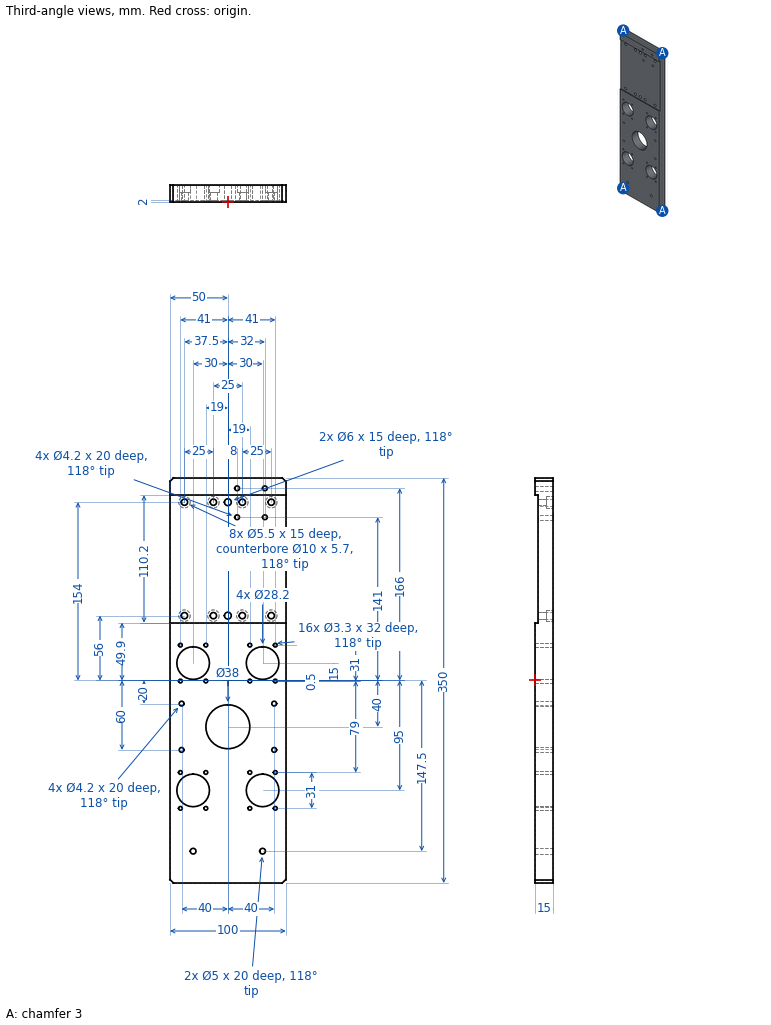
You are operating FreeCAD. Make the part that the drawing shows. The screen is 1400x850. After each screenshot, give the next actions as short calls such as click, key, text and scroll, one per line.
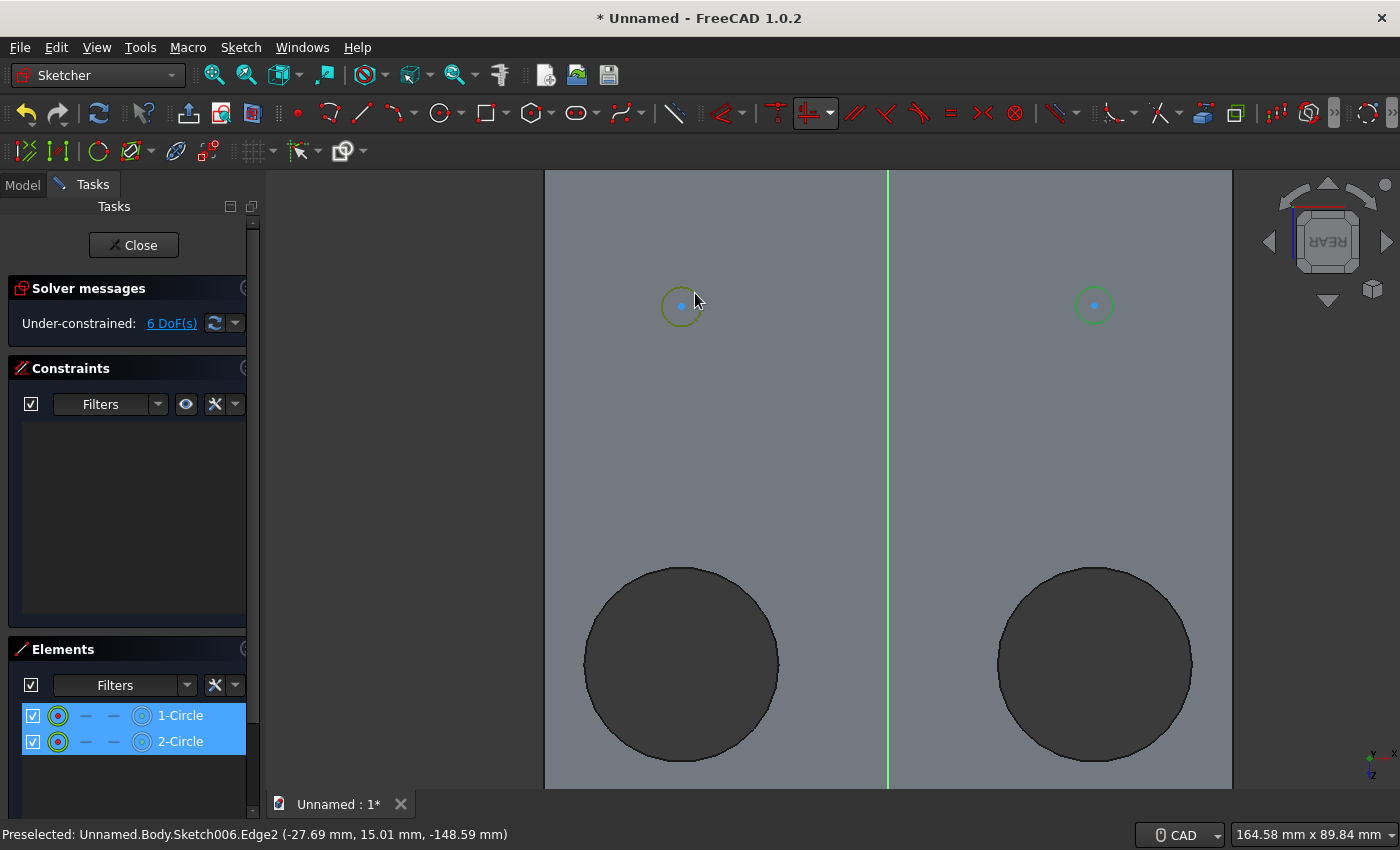
key(e)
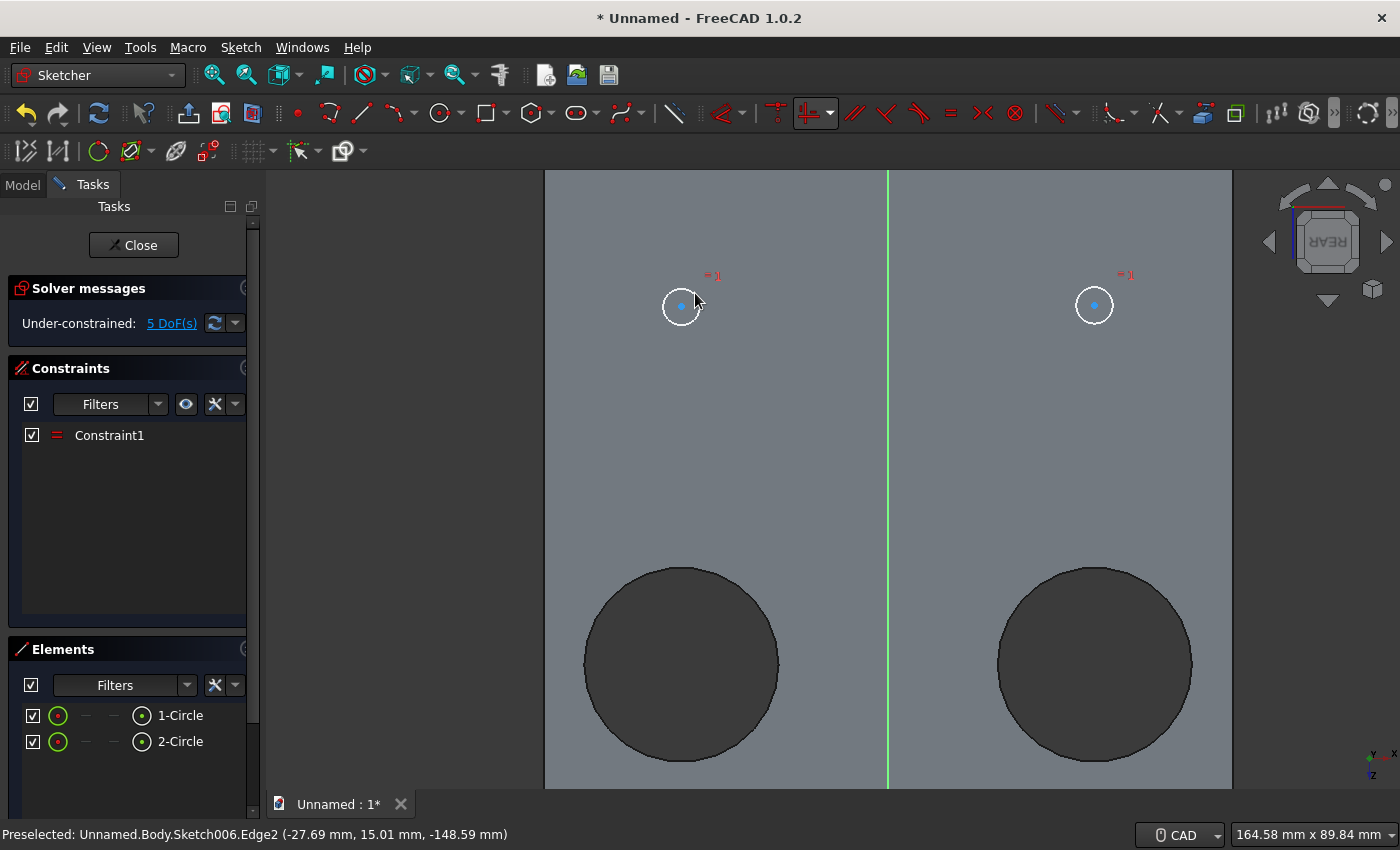
click(1094, 305)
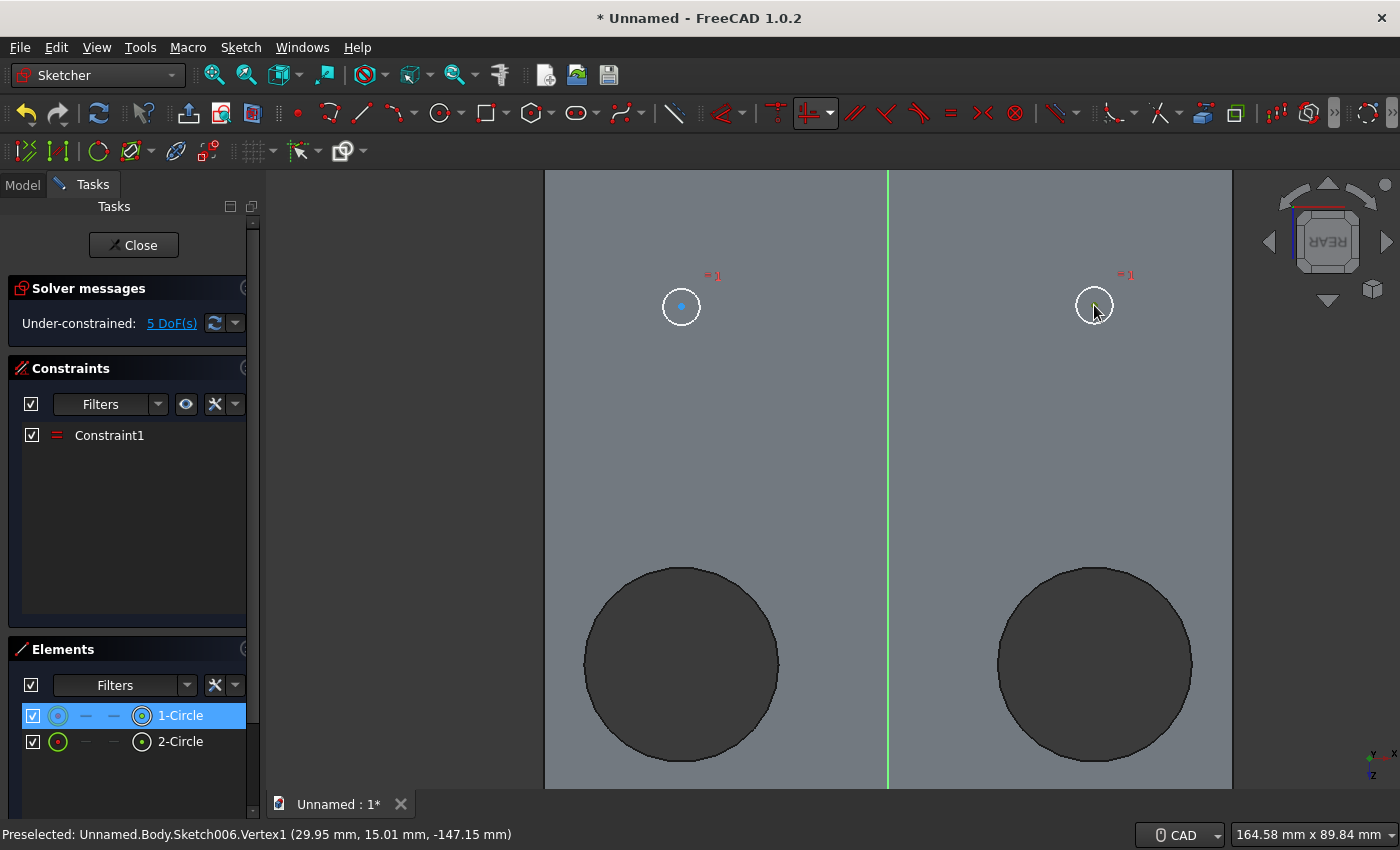
click(681, 307)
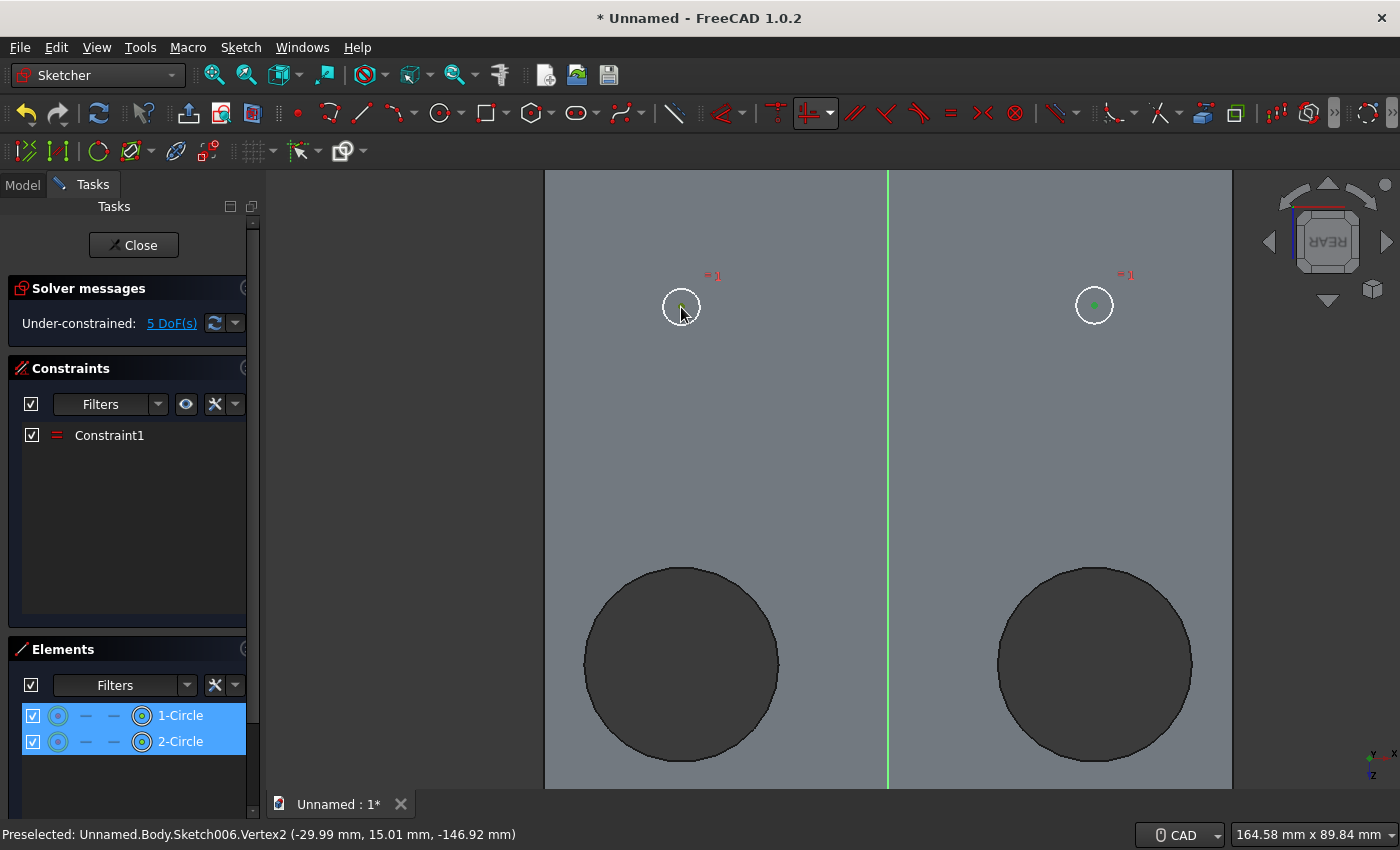
key(h)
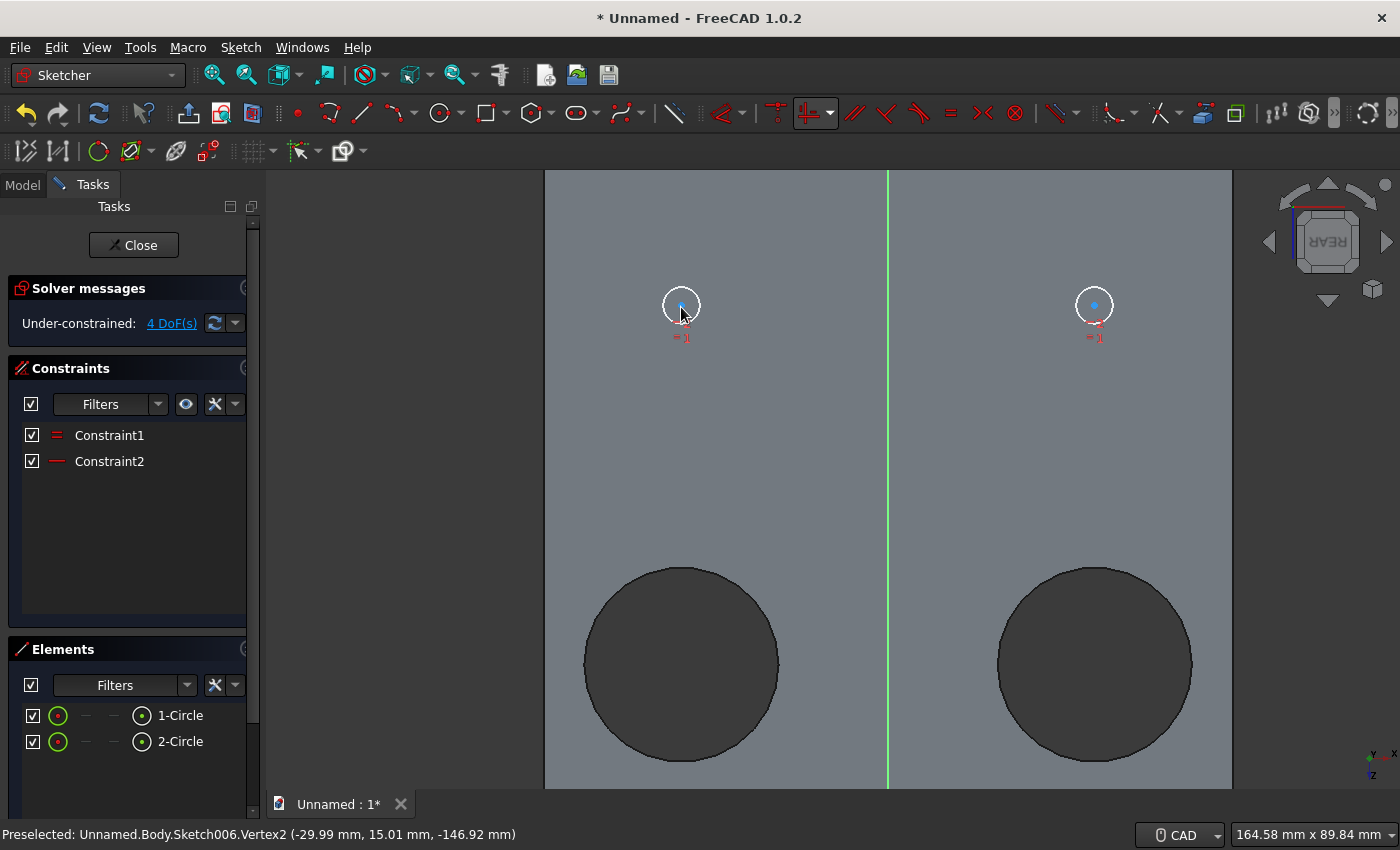
click(722, 114)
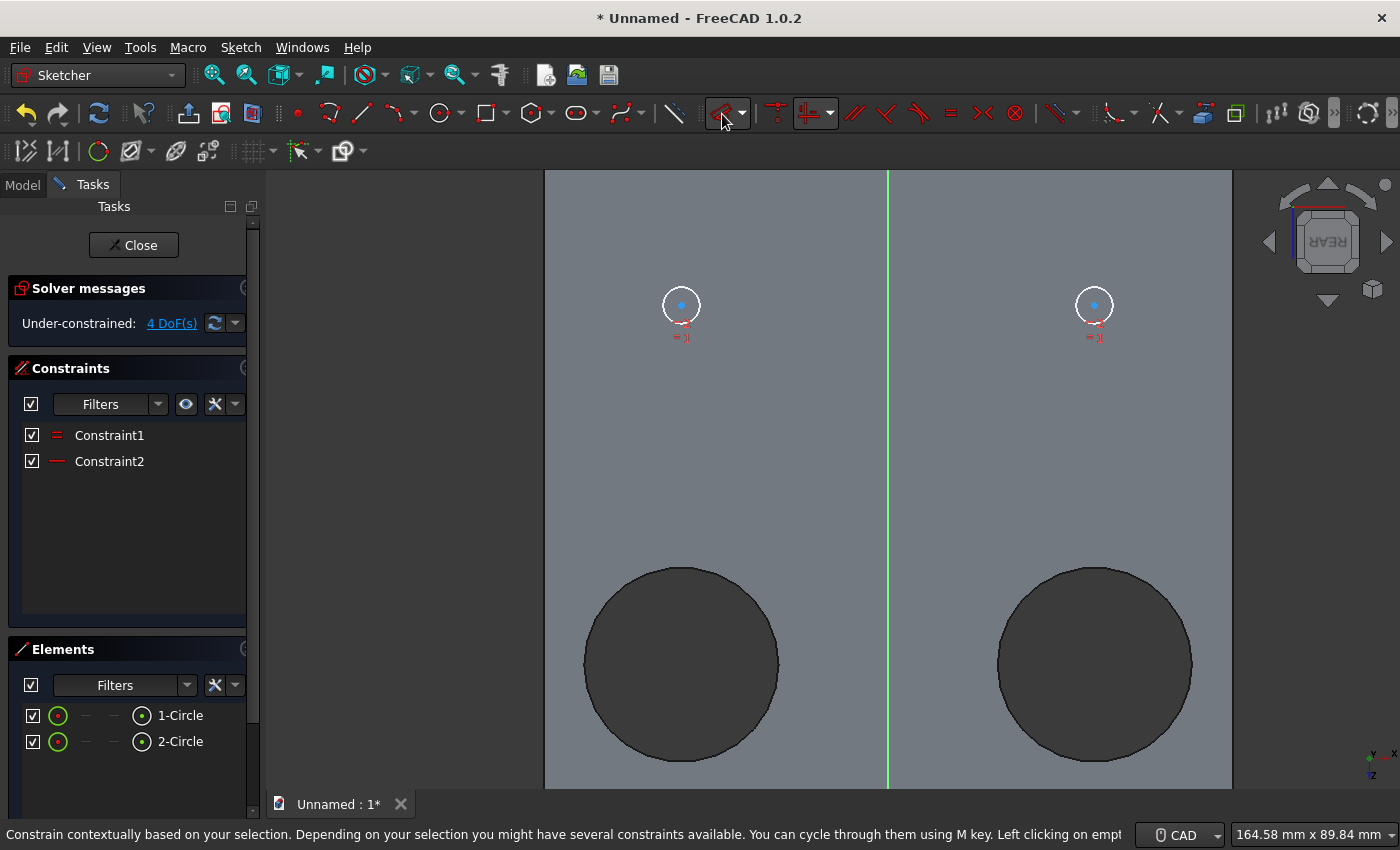
click(1107, 292)
click(1129, 269)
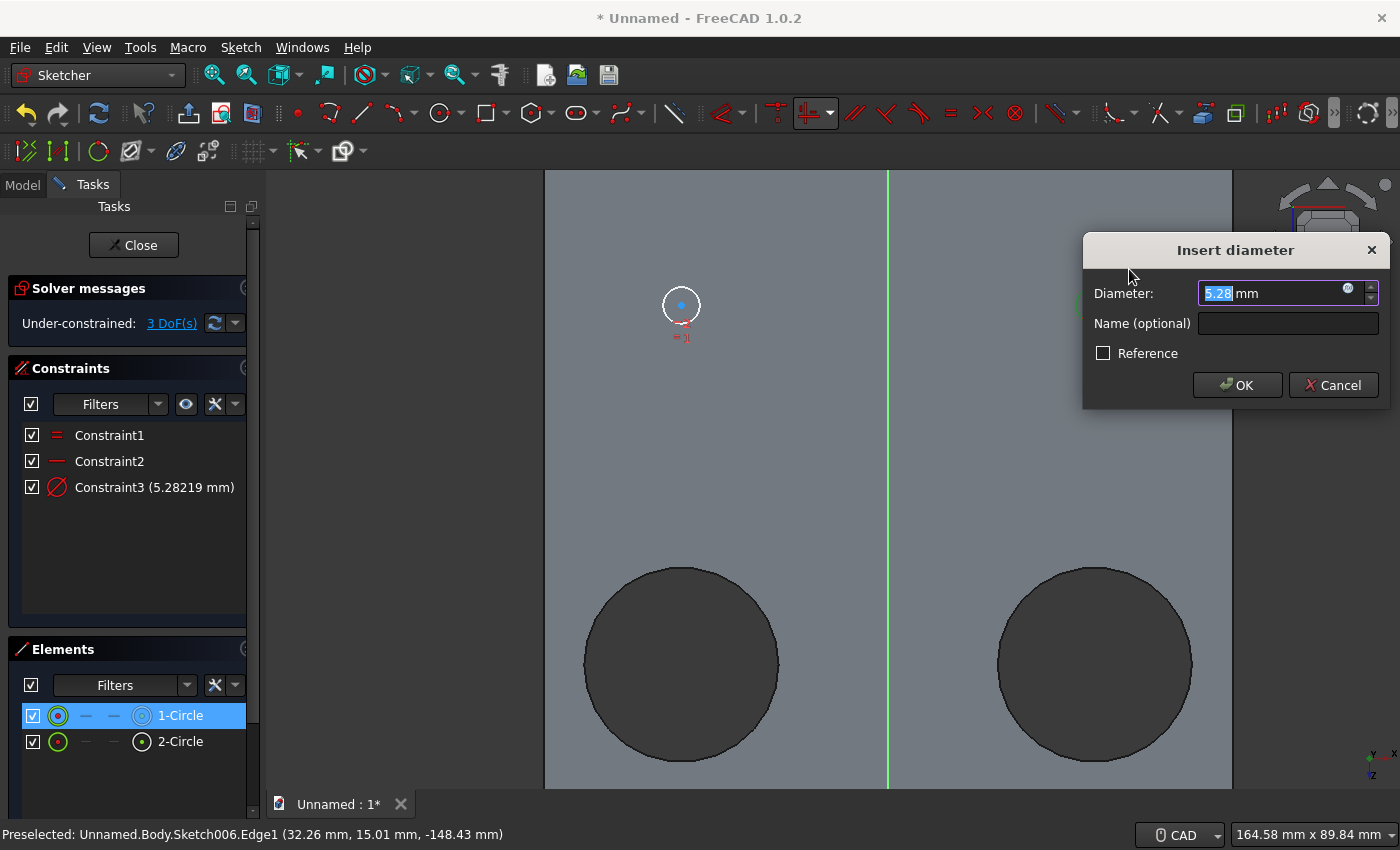
text(5)
key(Return)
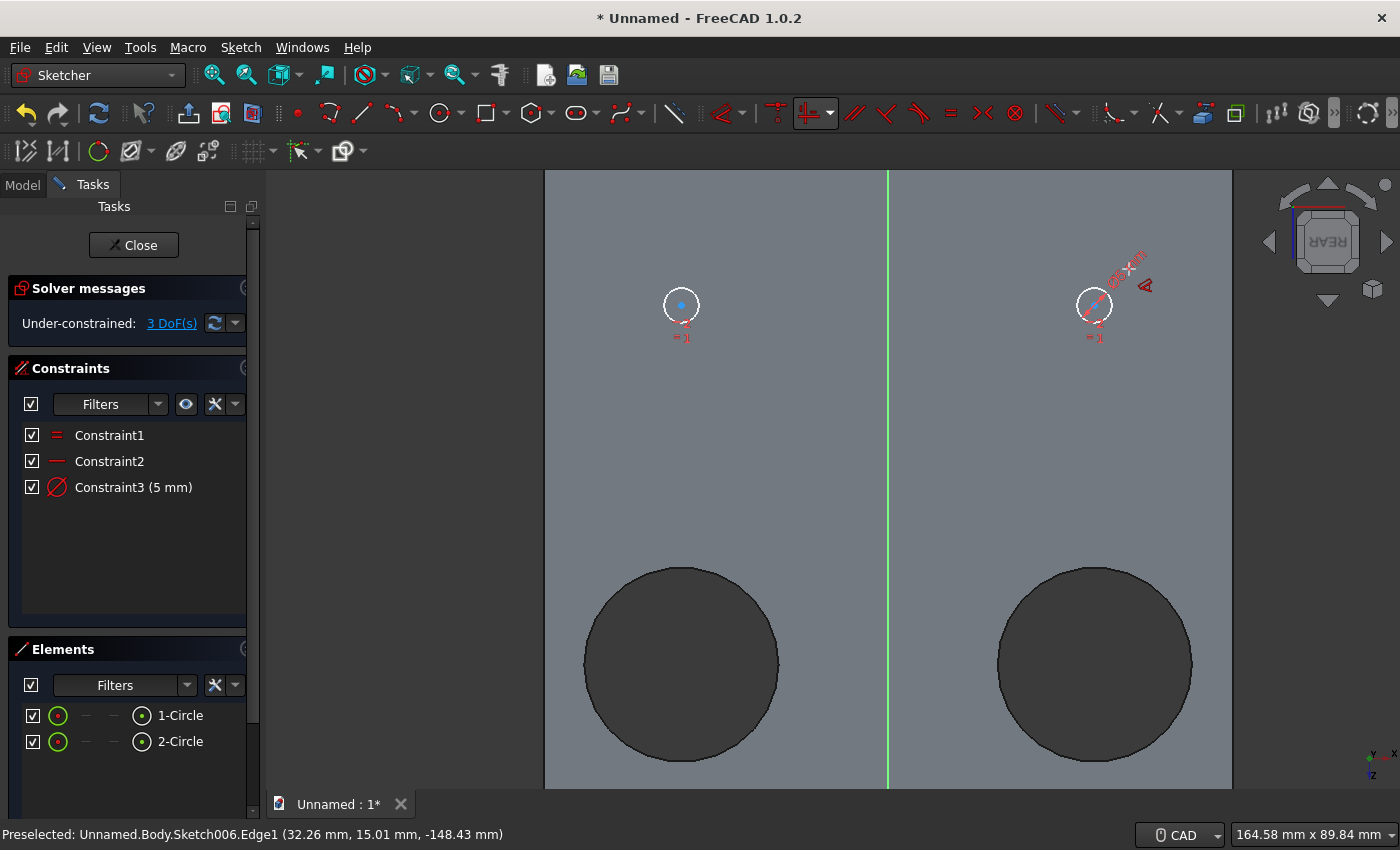
click(1094, 305)
click(991, 271)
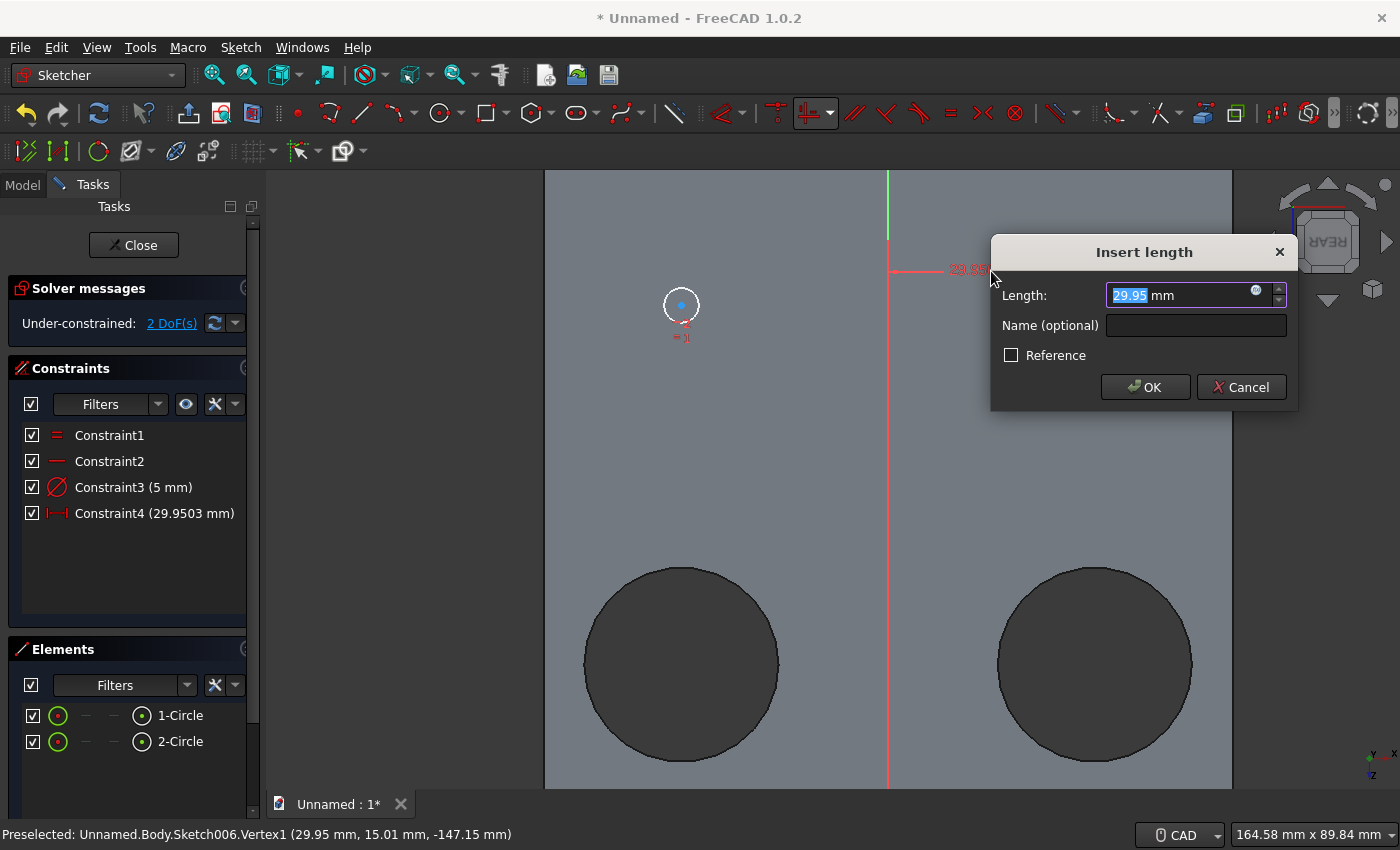
text(30)
key(Return)